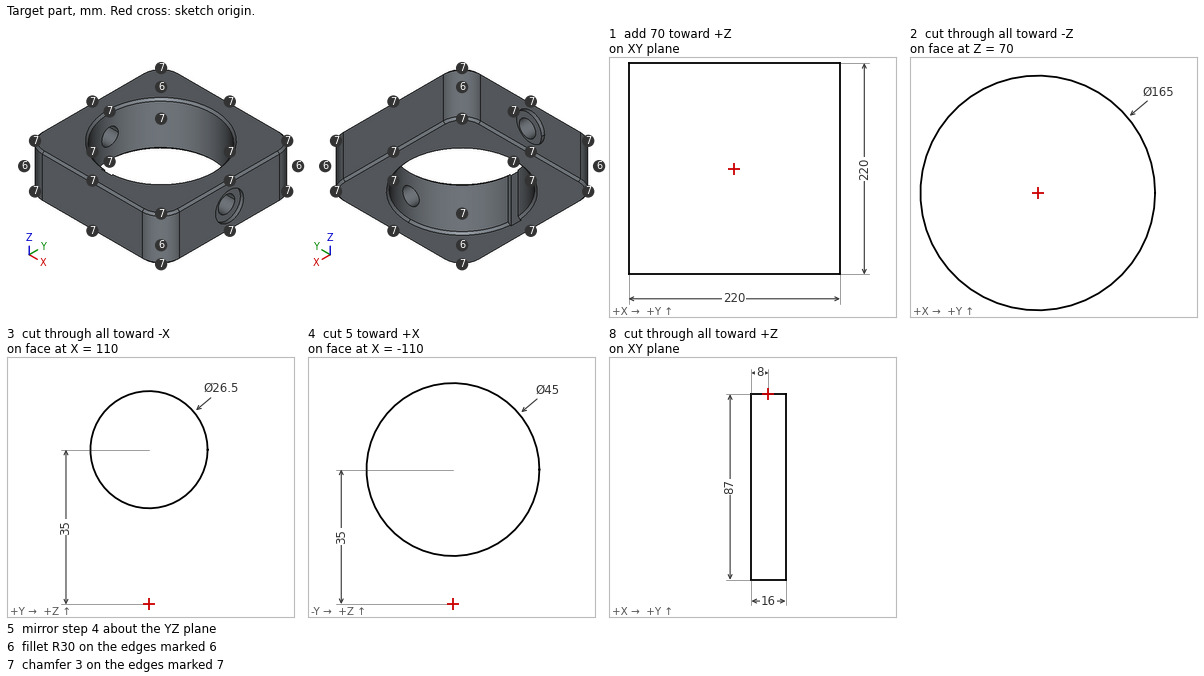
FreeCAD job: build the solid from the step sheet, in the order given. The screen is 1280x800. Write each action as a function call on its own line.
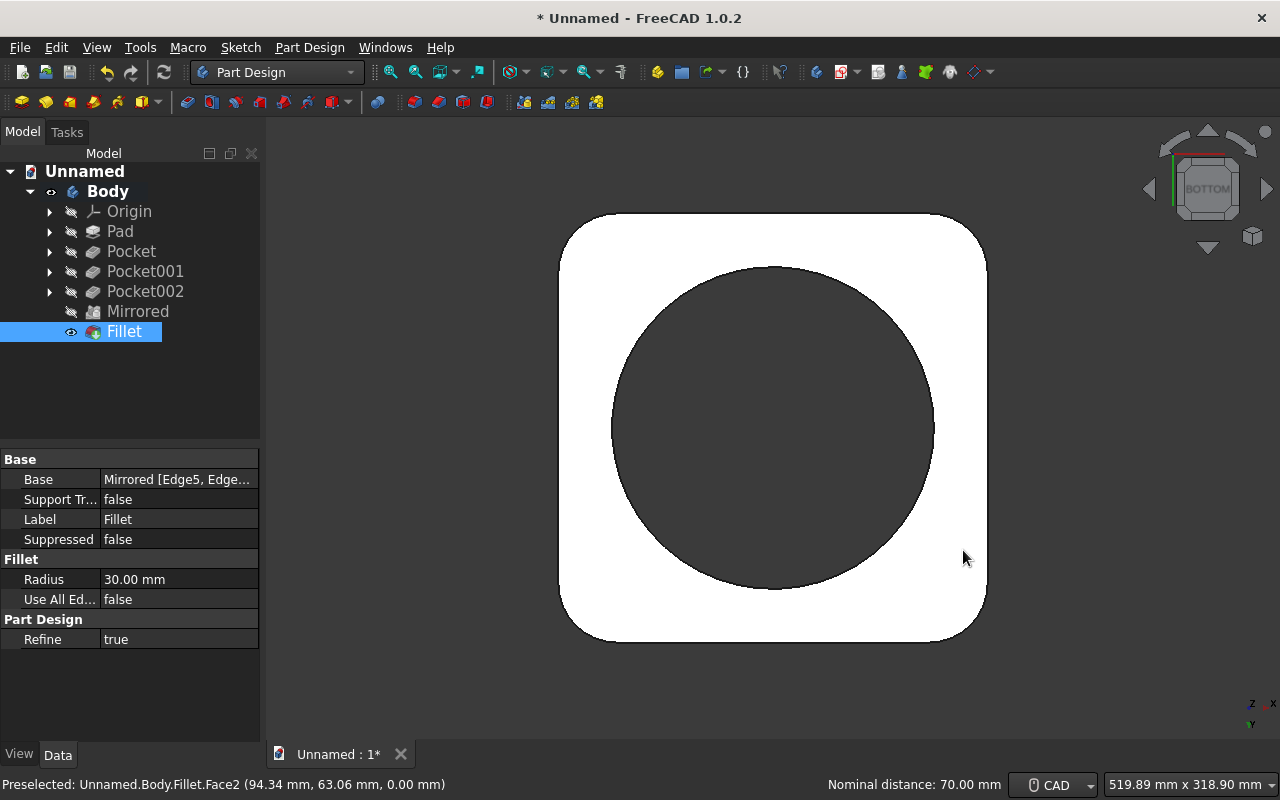
click(440, 102)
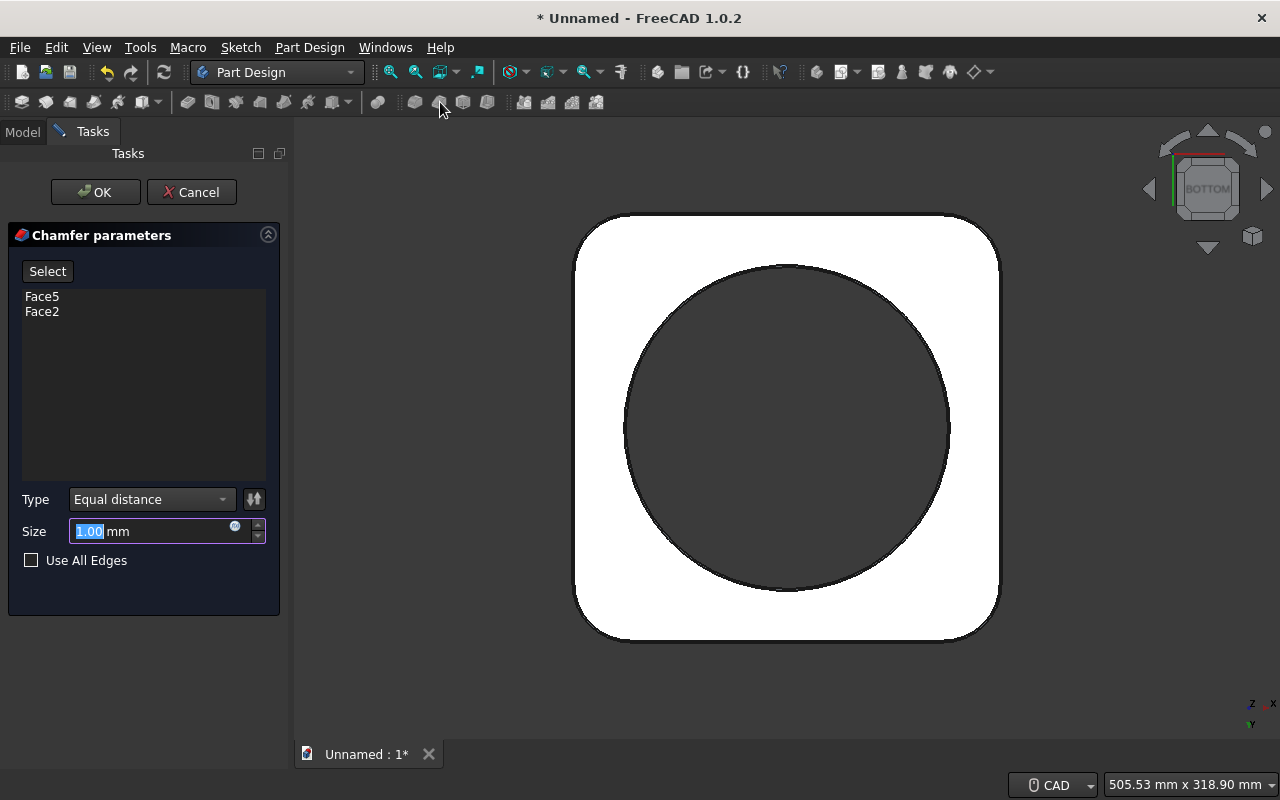
text(3)
key(Tab)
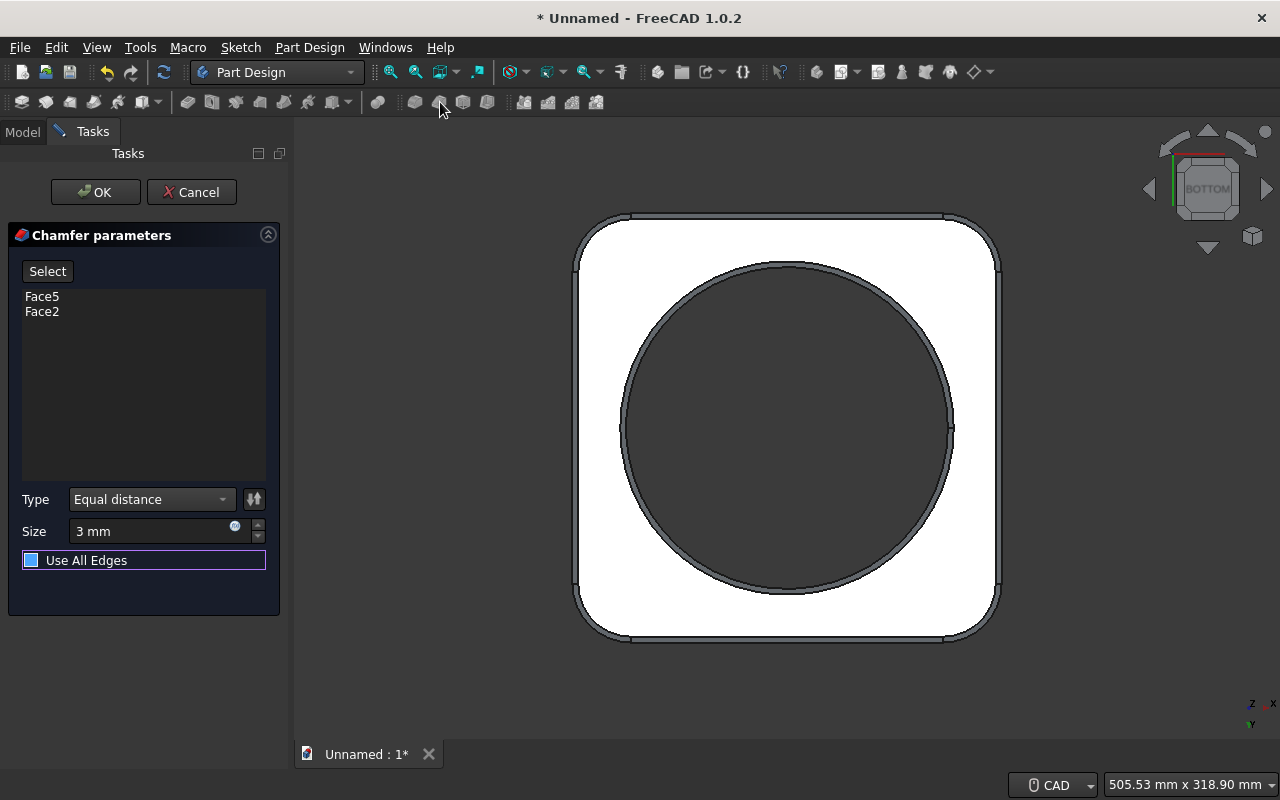
click(96, 192)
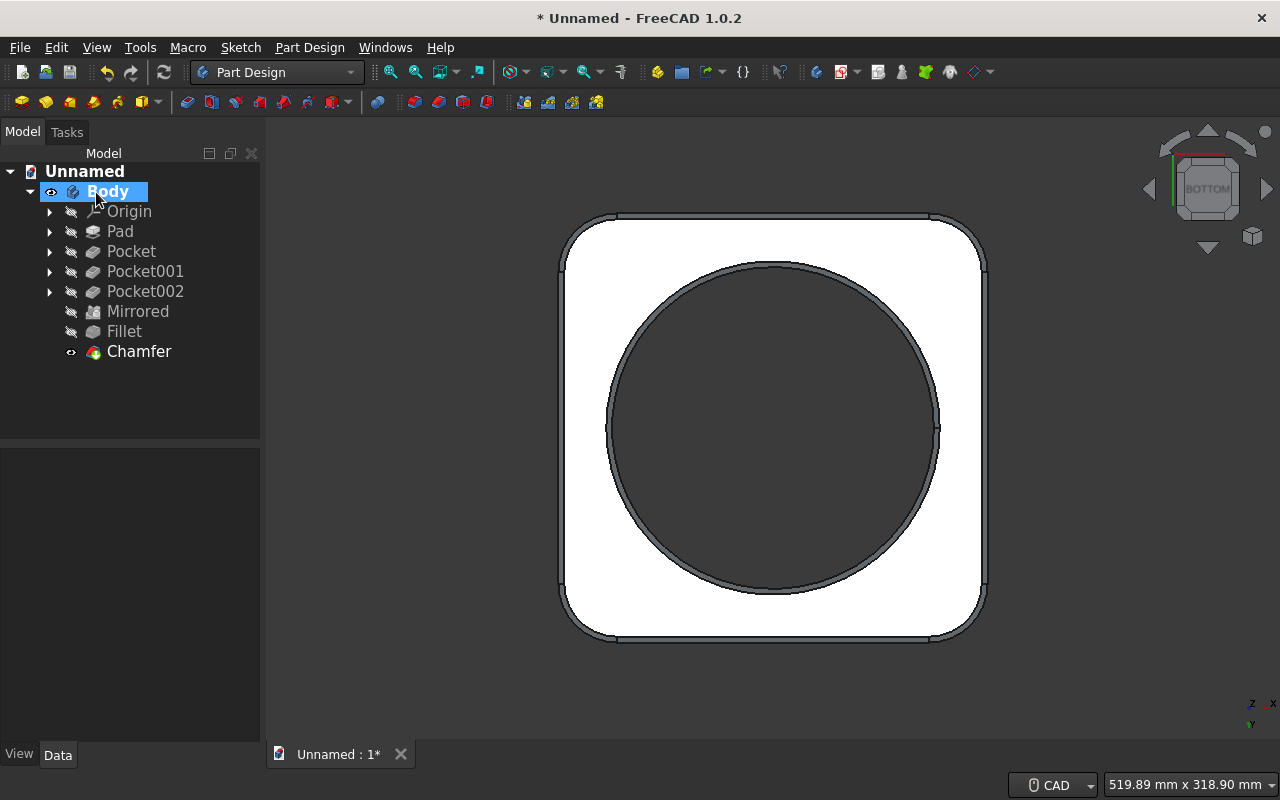
click(842, 72)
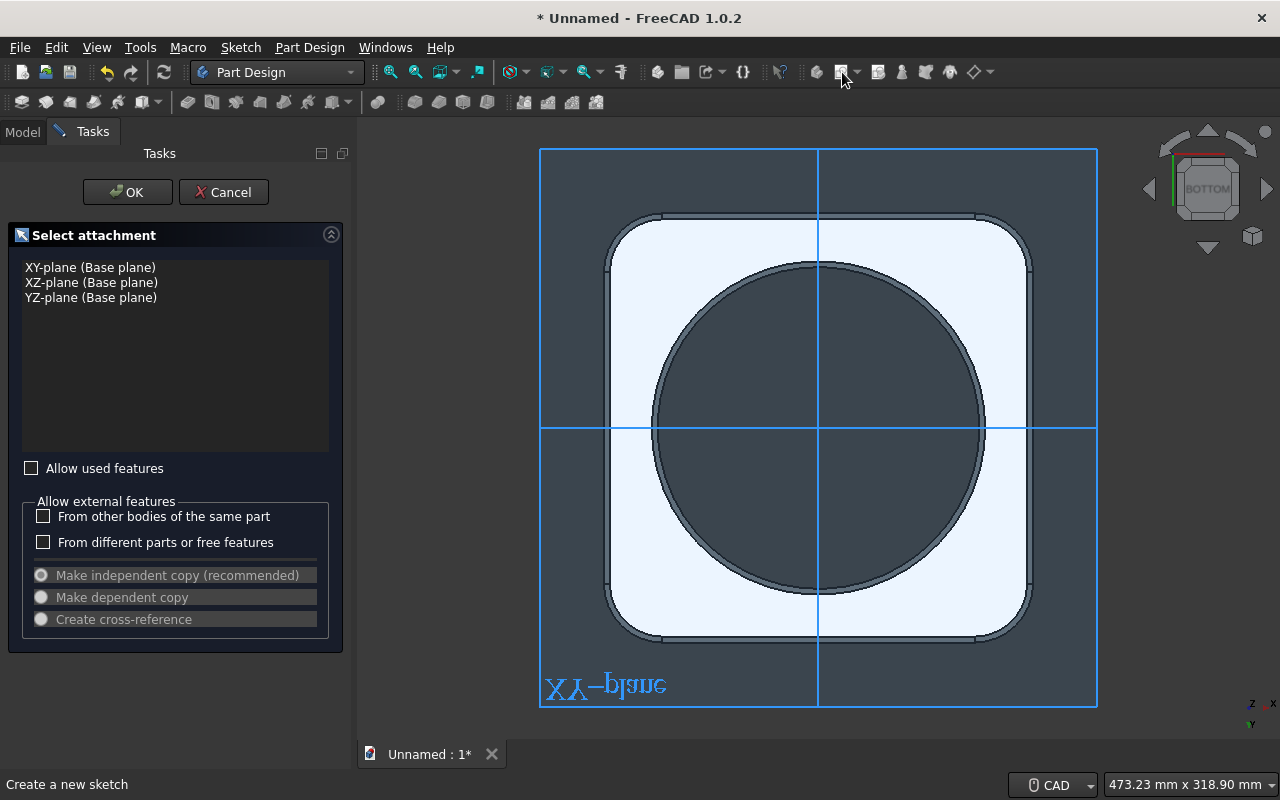
click(82, 268)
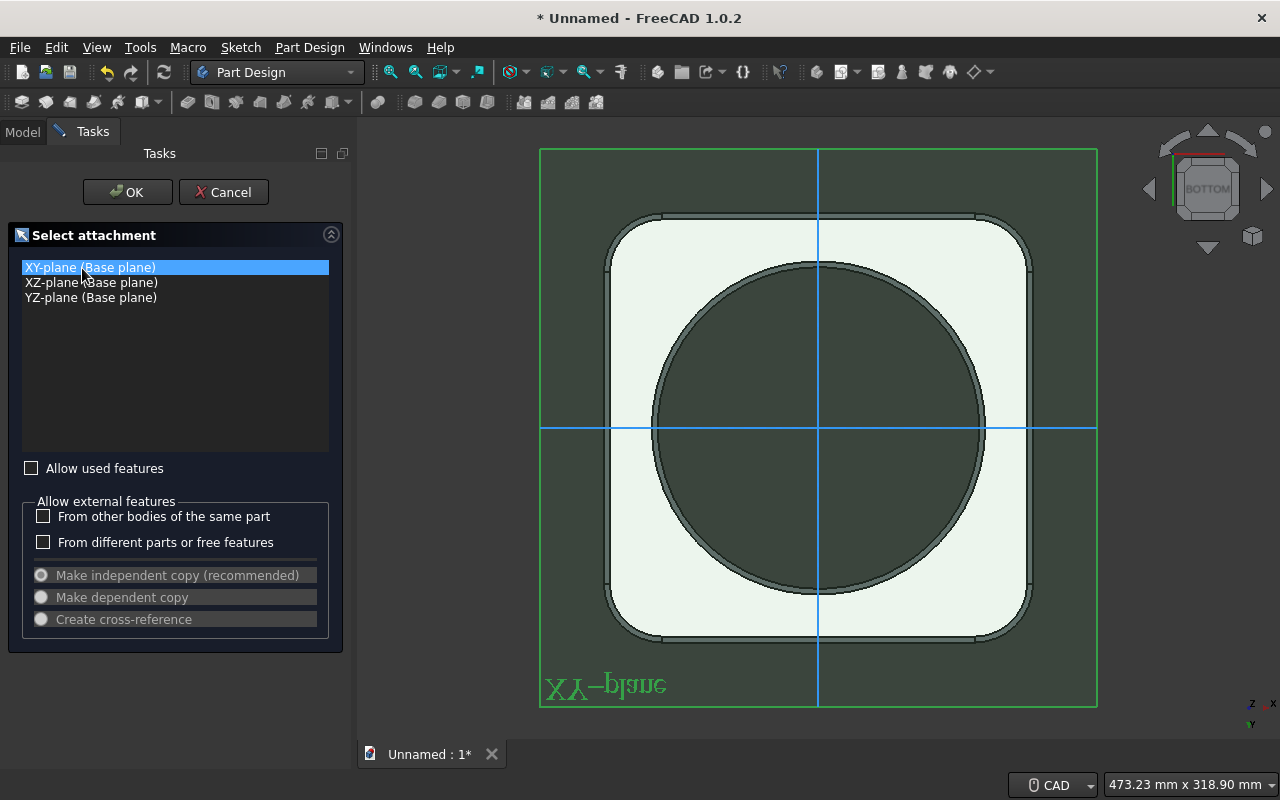
click(128, 192)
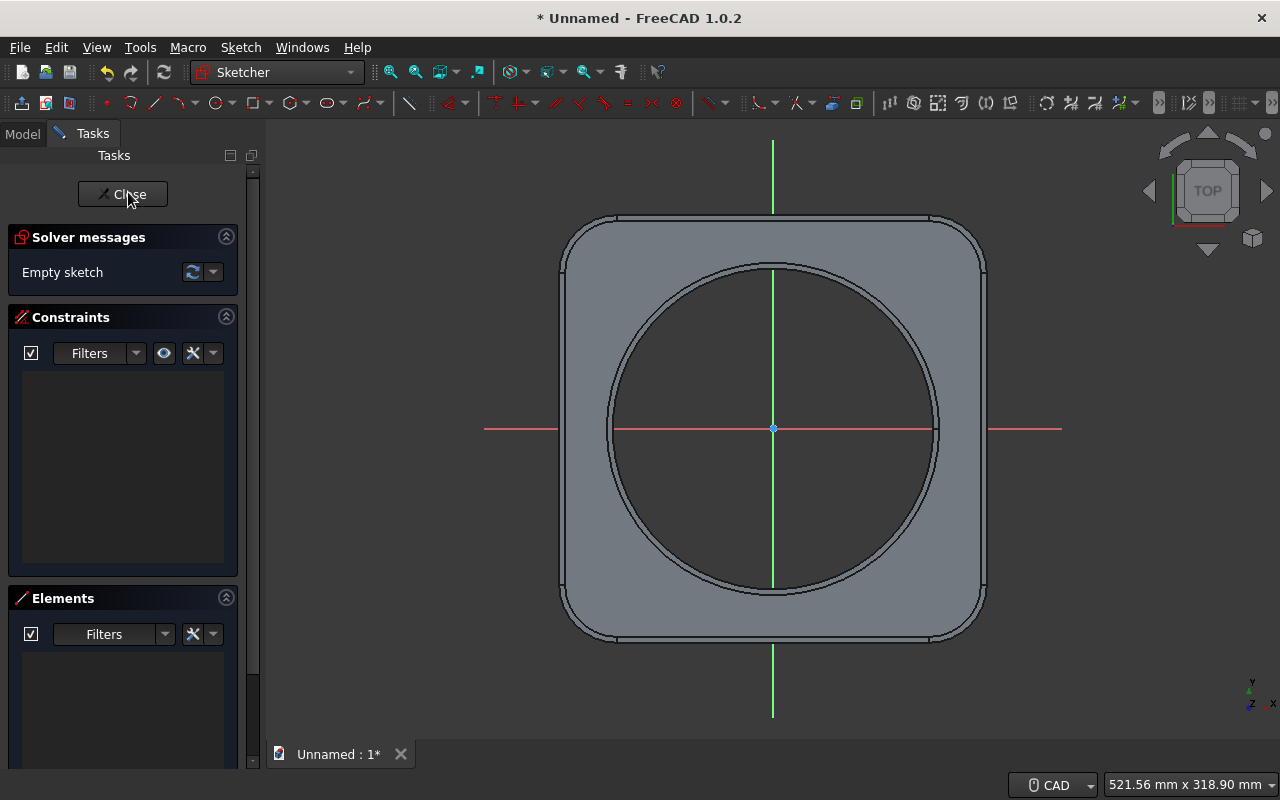
key(q)
key(s)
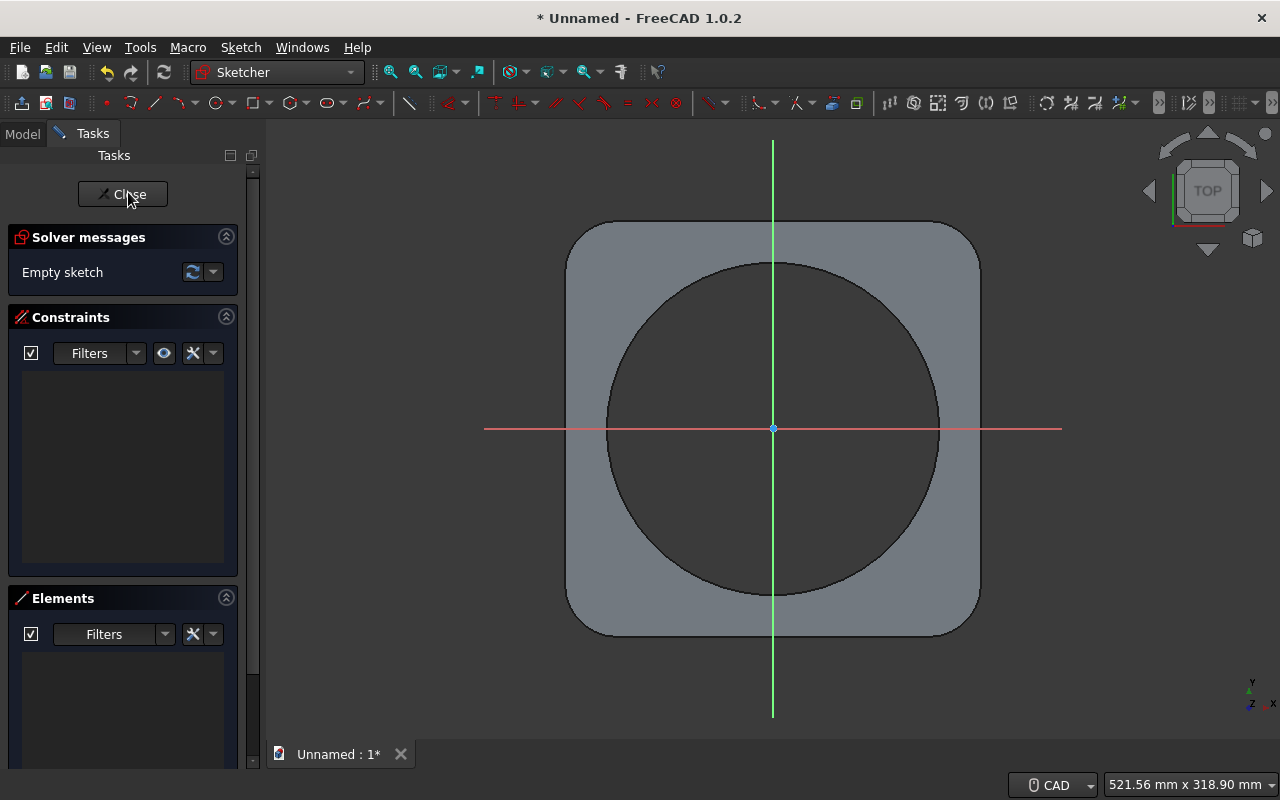
scroll(829, 583, up, 4)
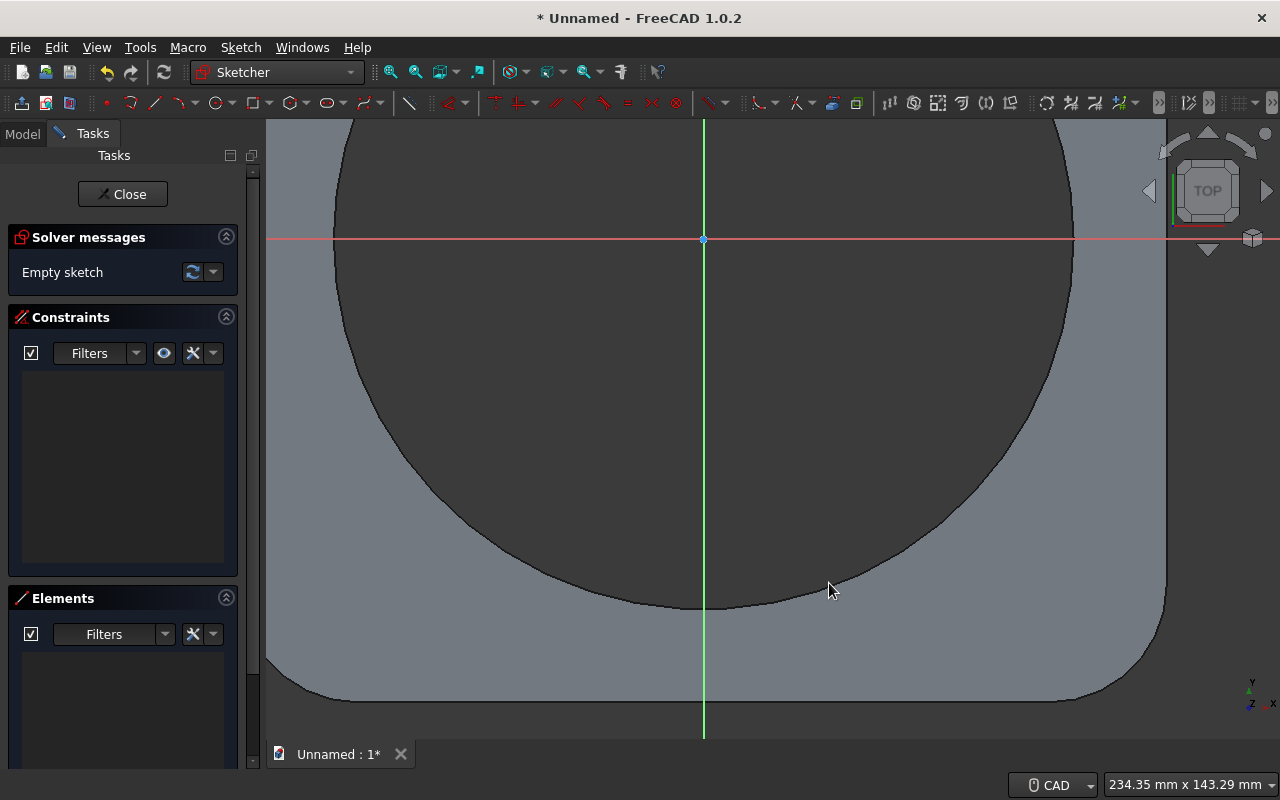
key(g)
key(r)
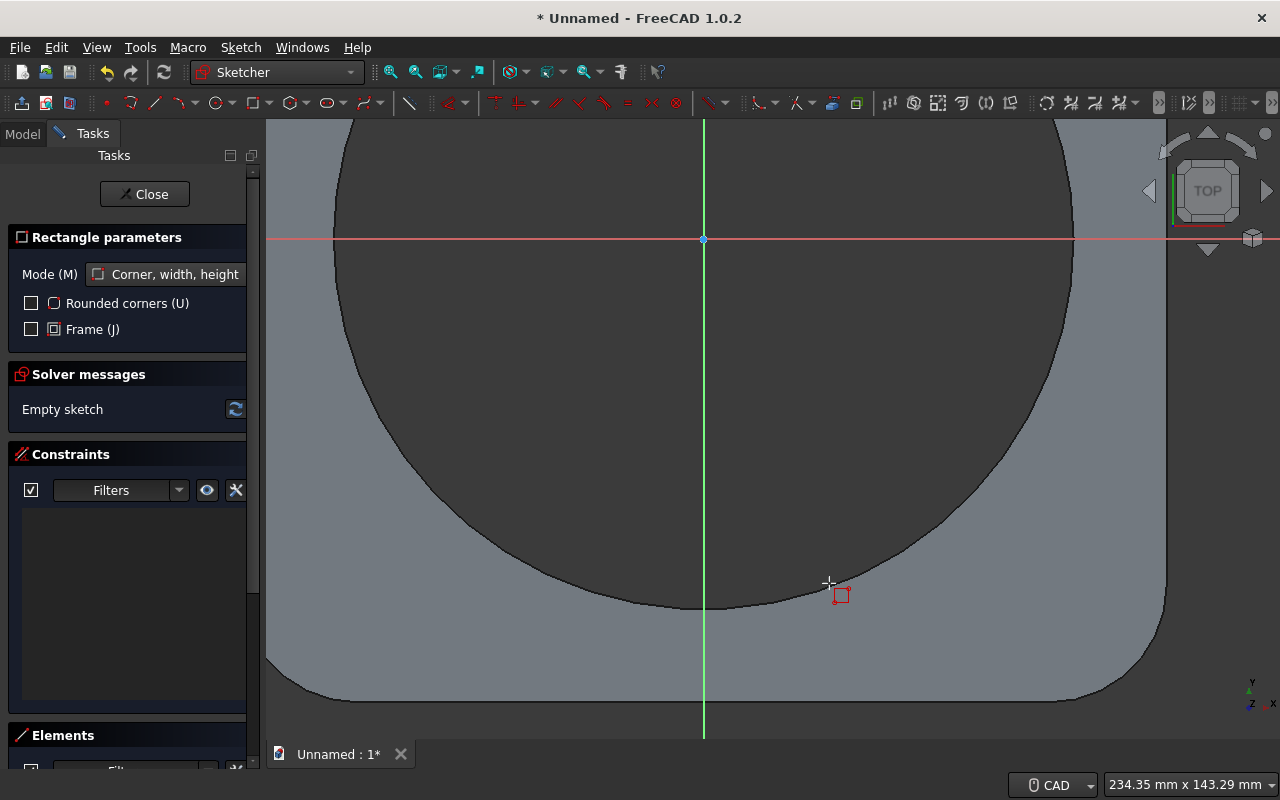
click(669, 239)
click(738, 616)
key(Escape)